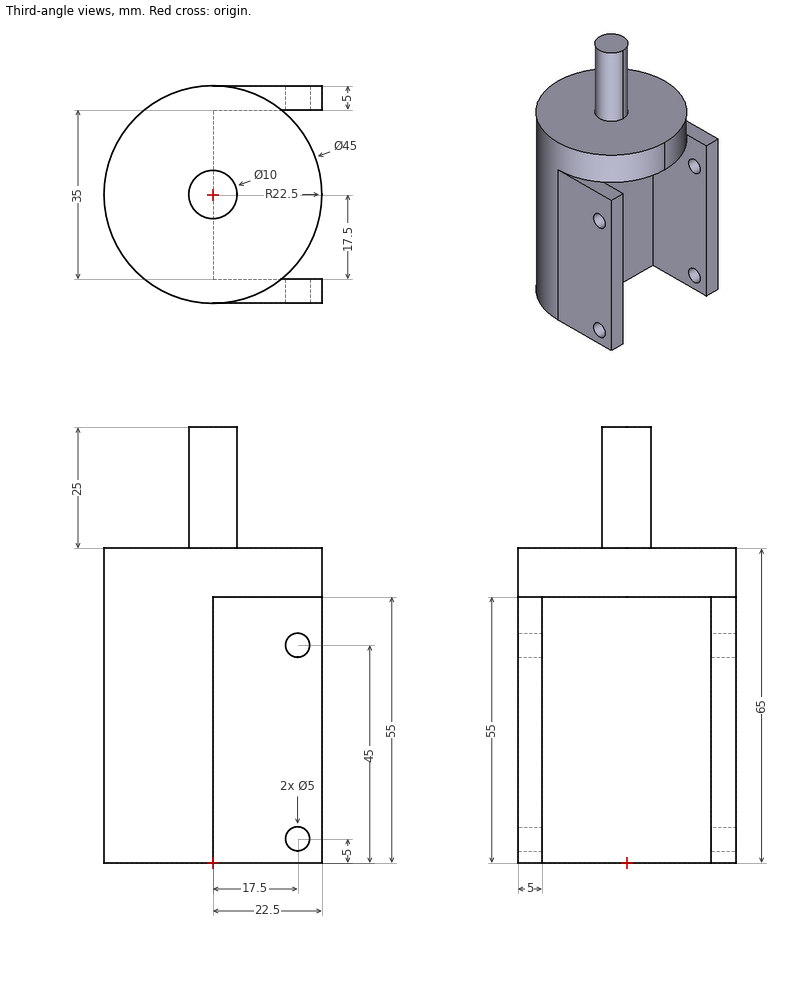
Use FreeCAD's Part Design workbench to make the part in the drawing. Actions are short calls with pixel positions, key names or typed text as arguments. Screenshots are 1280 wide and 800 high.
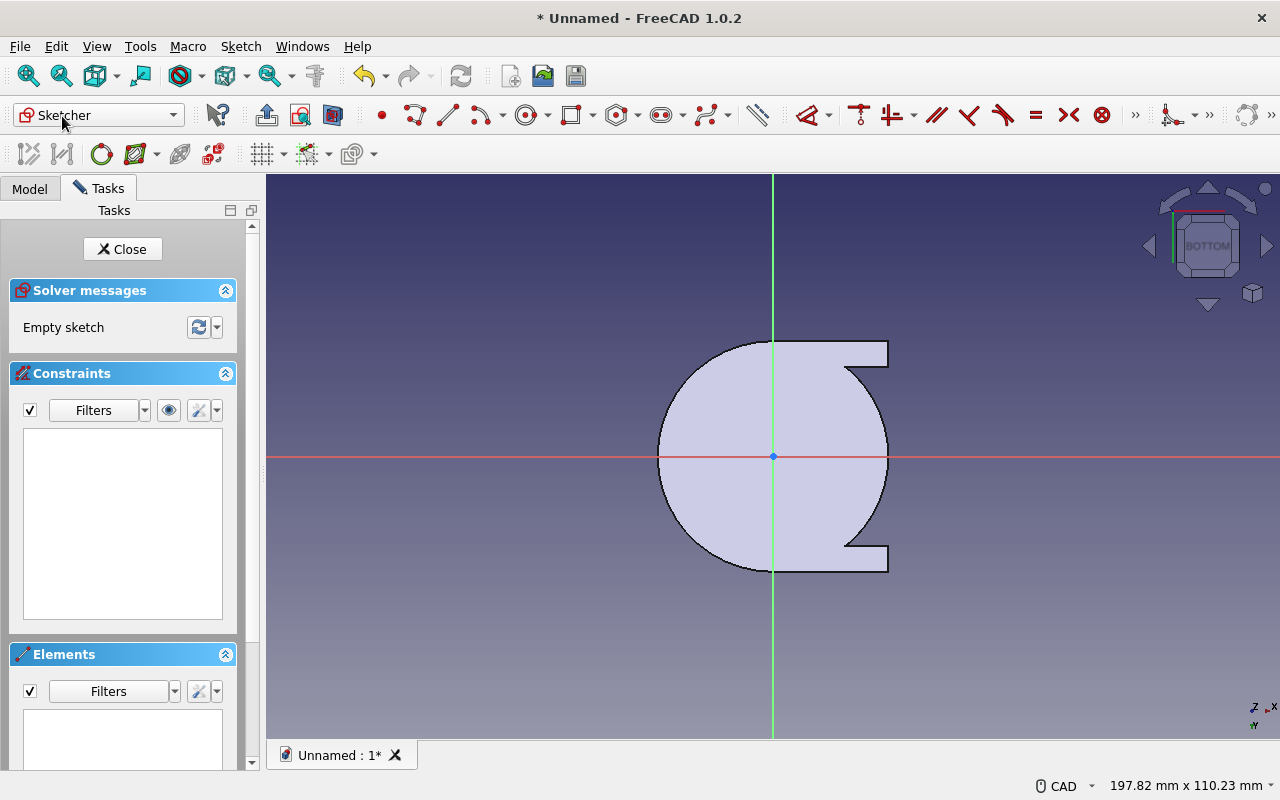
scroll(984, 456, up, 3)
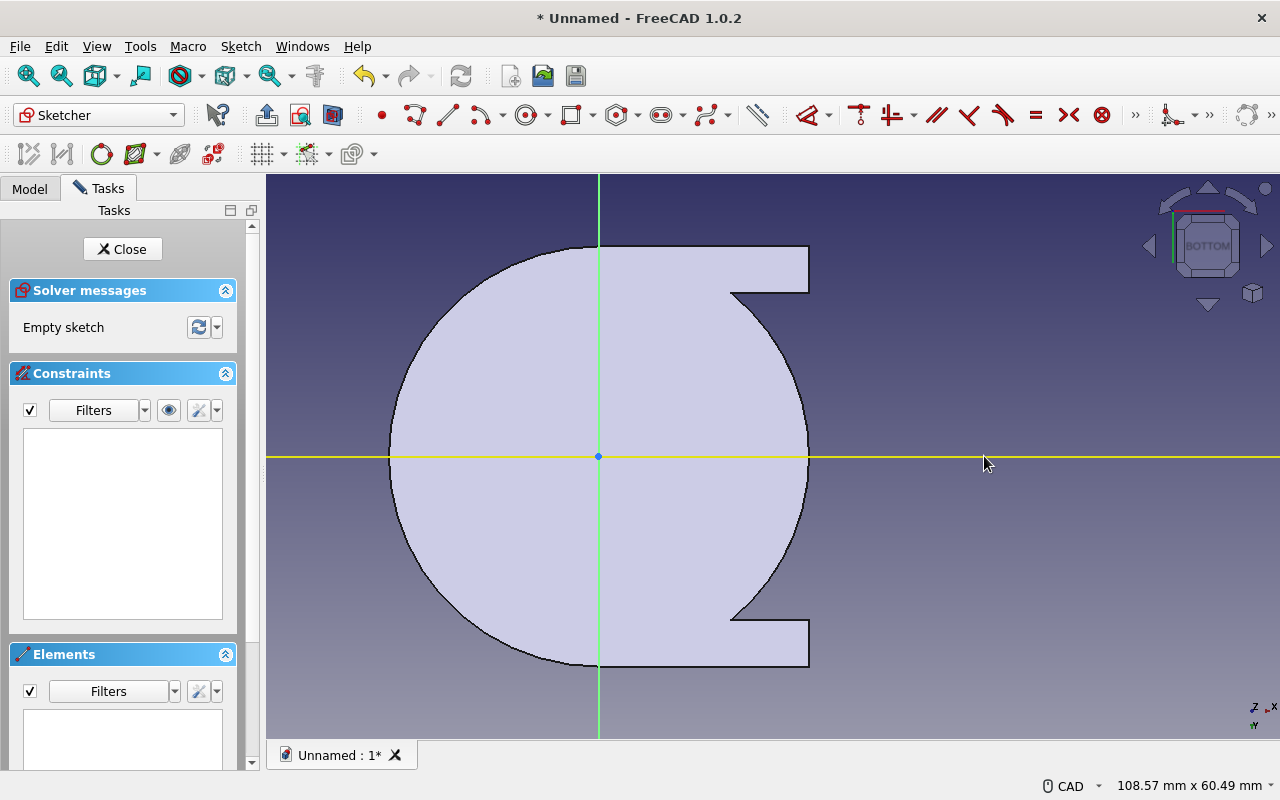
click(415, 116)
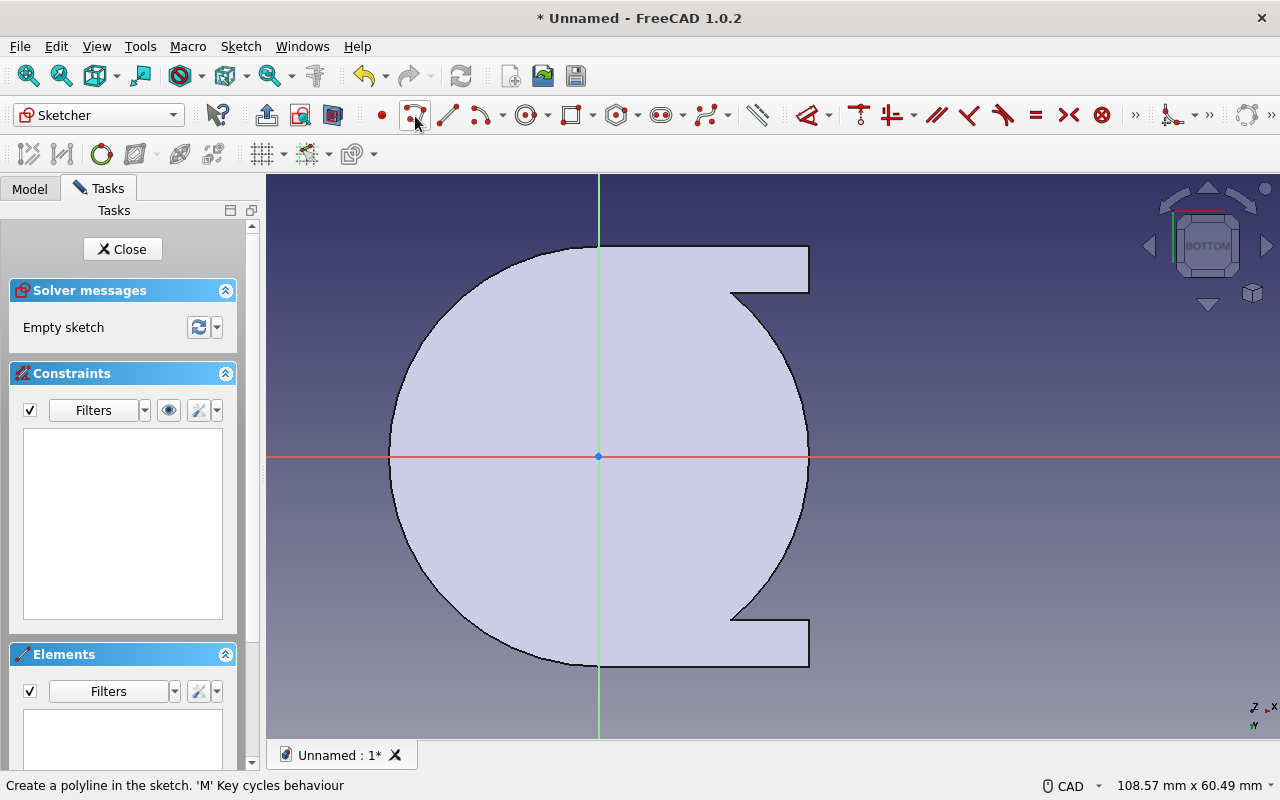
click(731, 293)
click(599, 293)
click(608, 620)
click(731, 620)
right_click(731, 620)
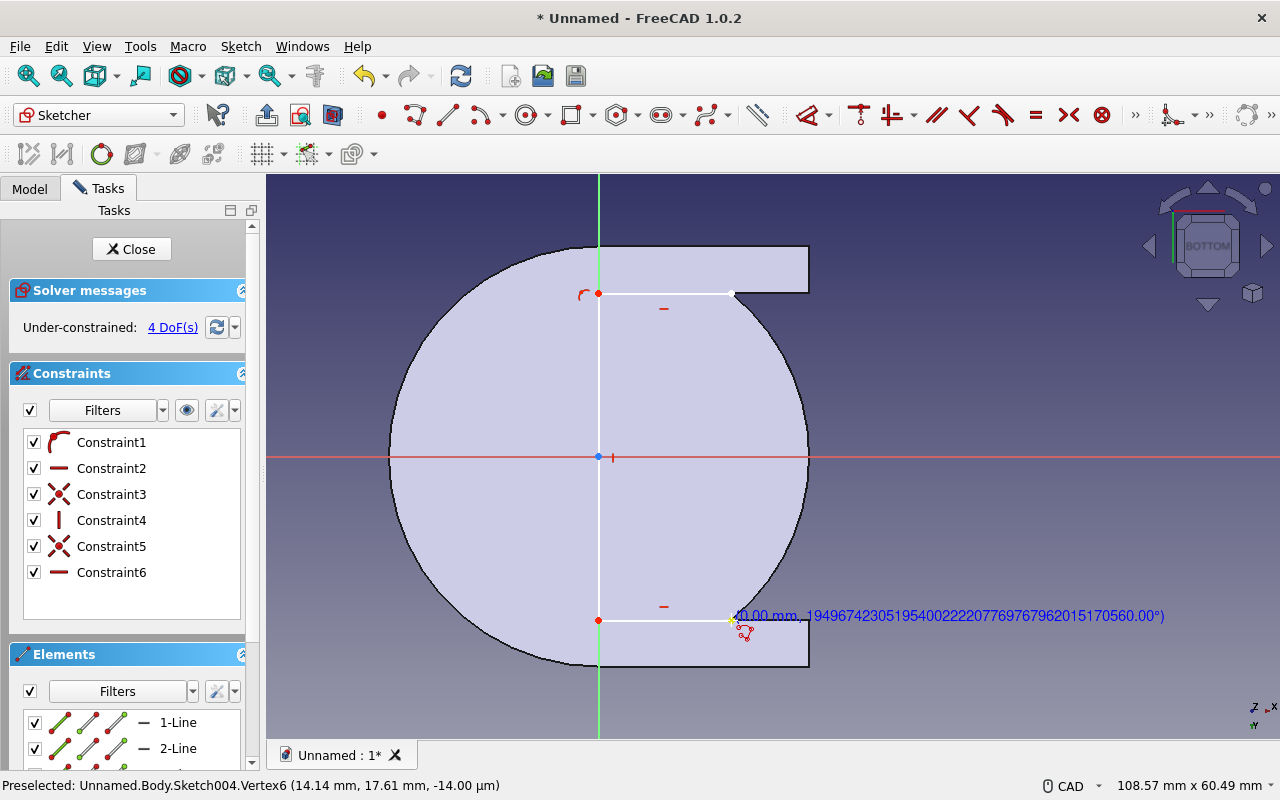
key(g)
key(3)
key(a)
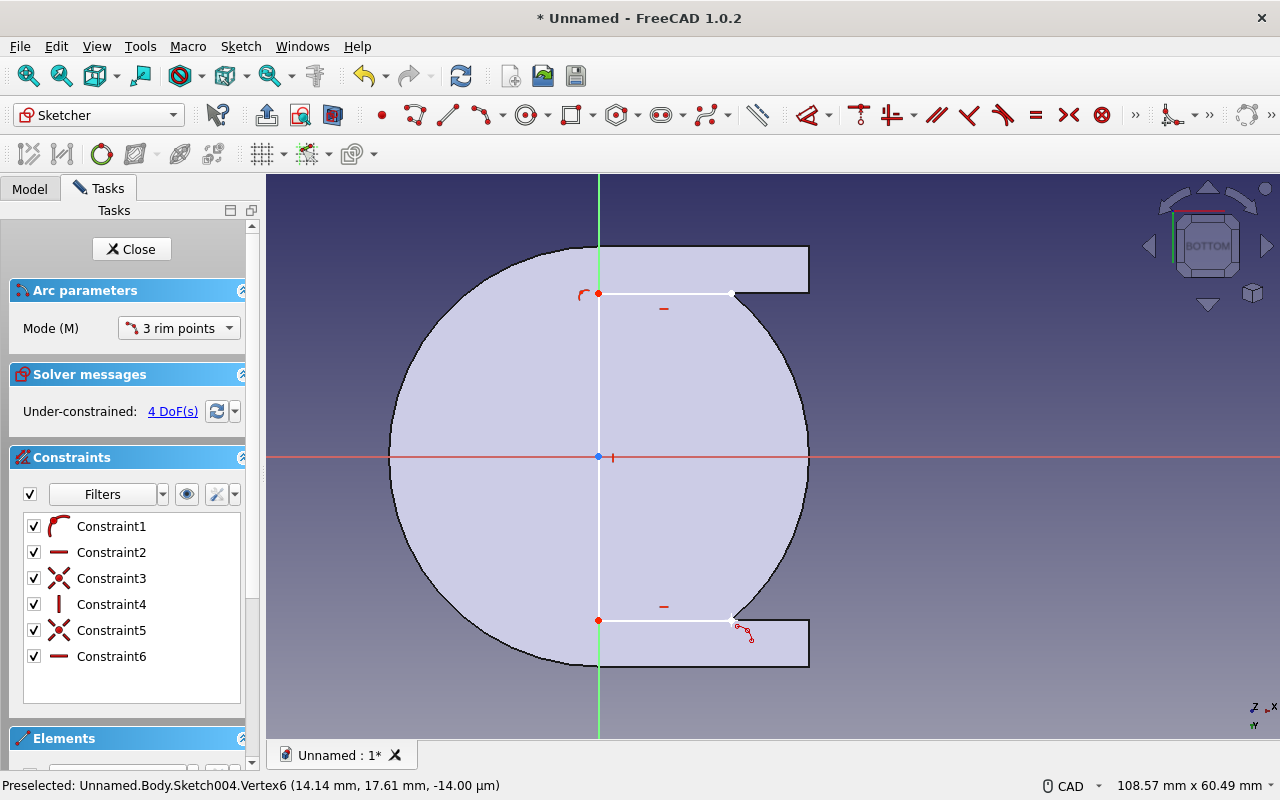
click(731, 621)
click(731, 294)
click(806, 494)
key(Escape)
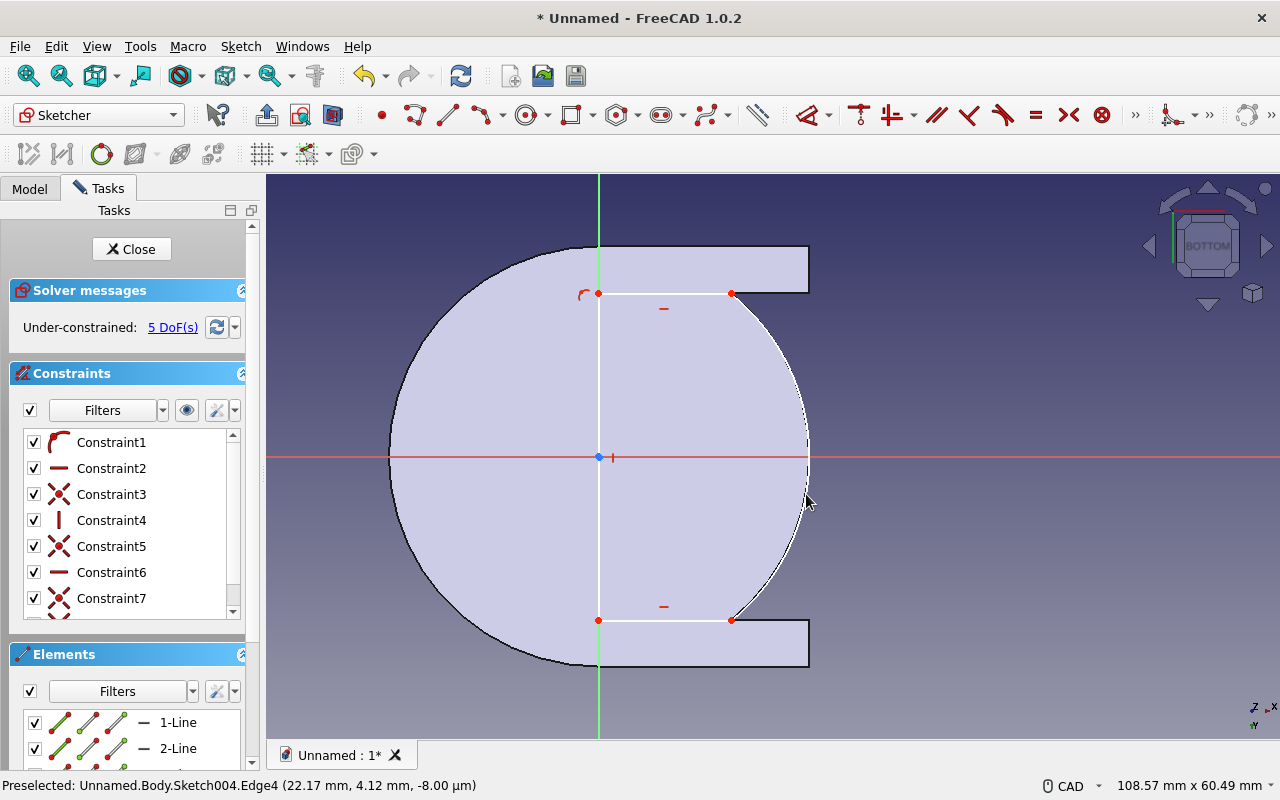
drag(589, 446, 610, 468)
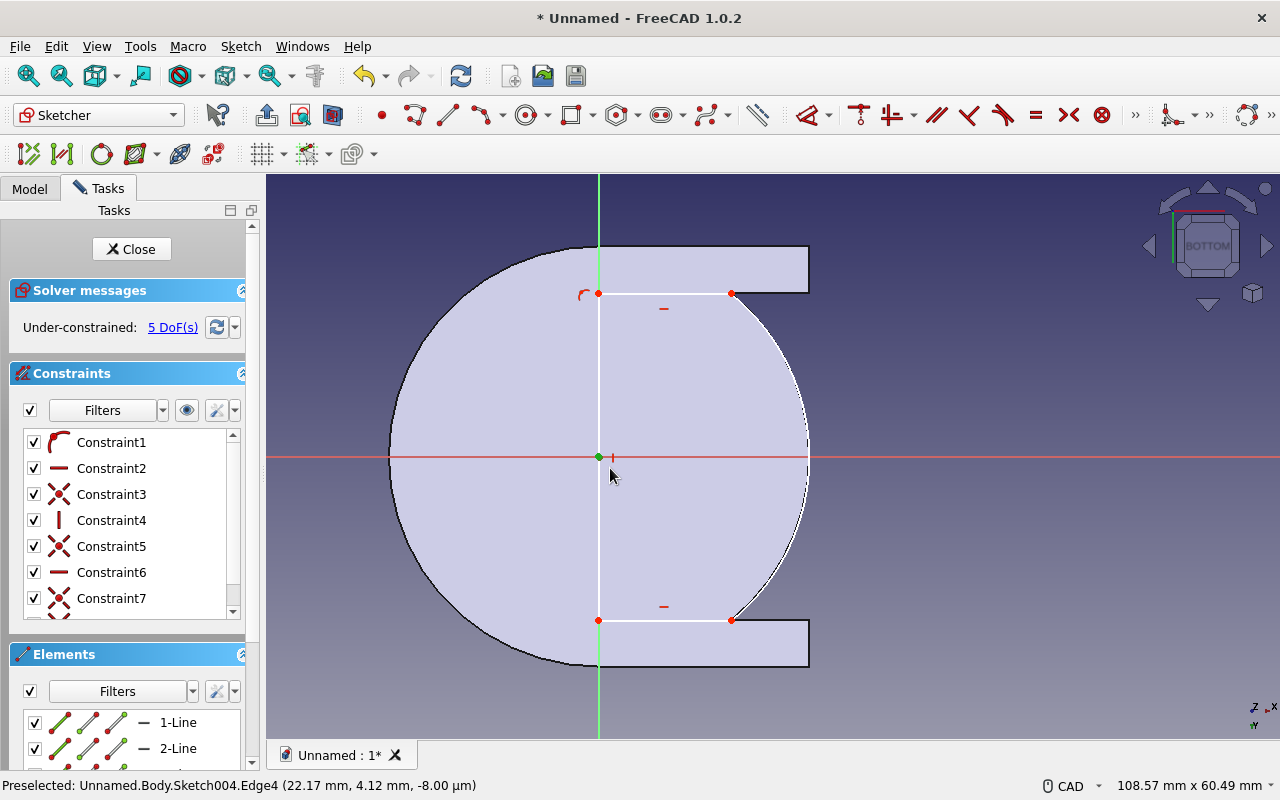
click(859, 116)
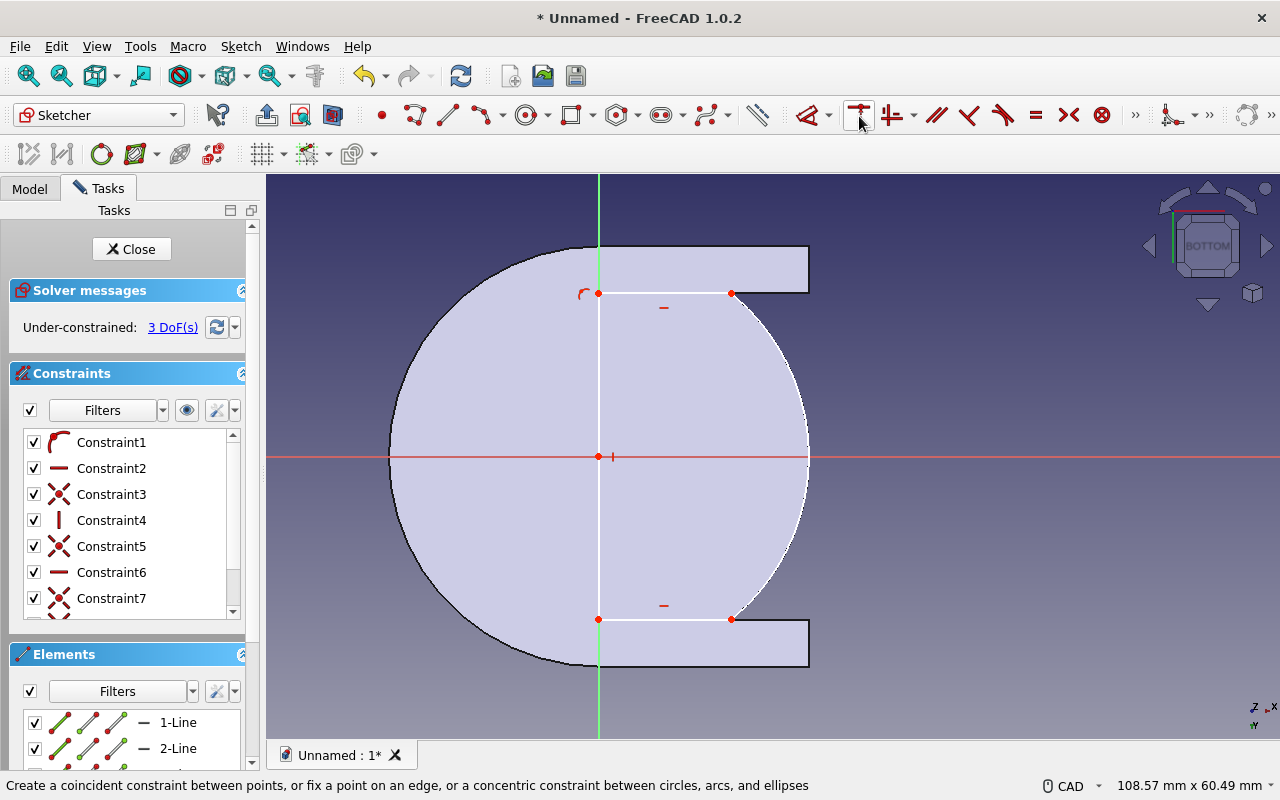
click(806, 116)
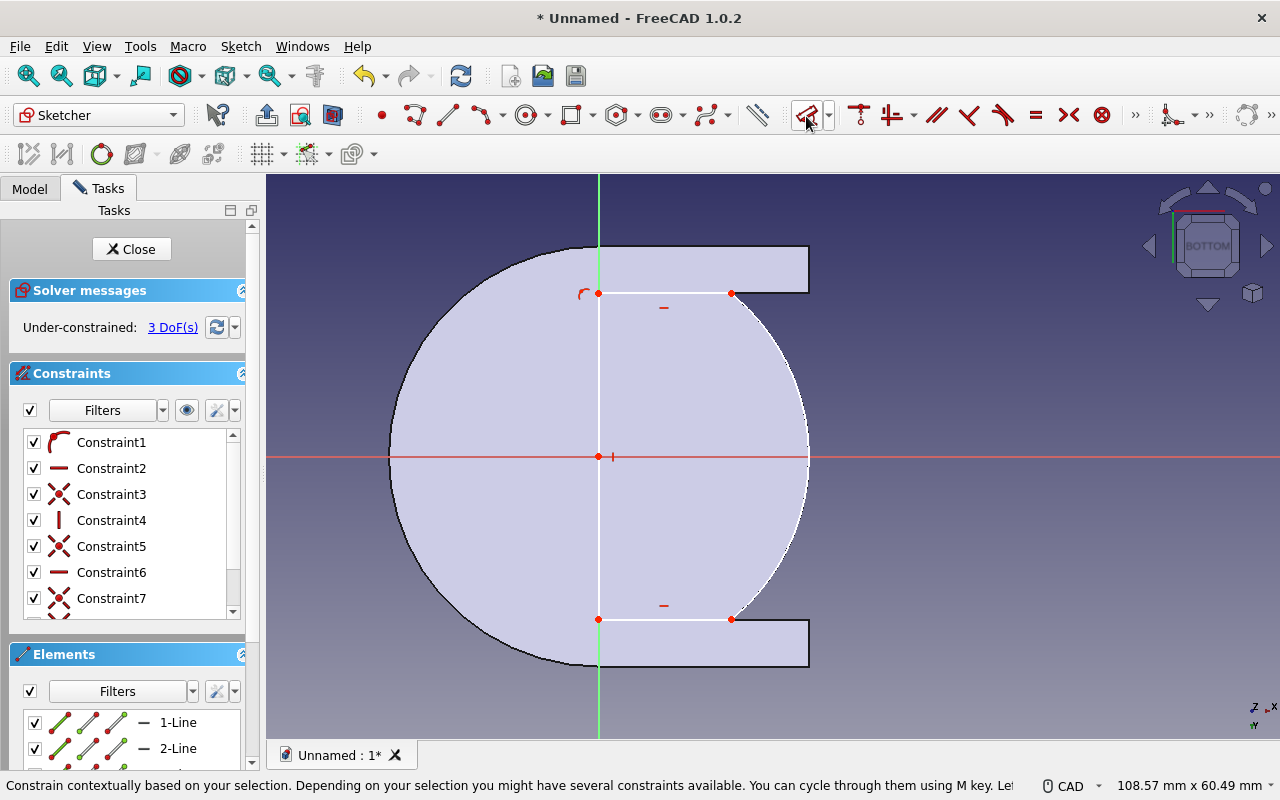
click(796, 530)
click(826, 541)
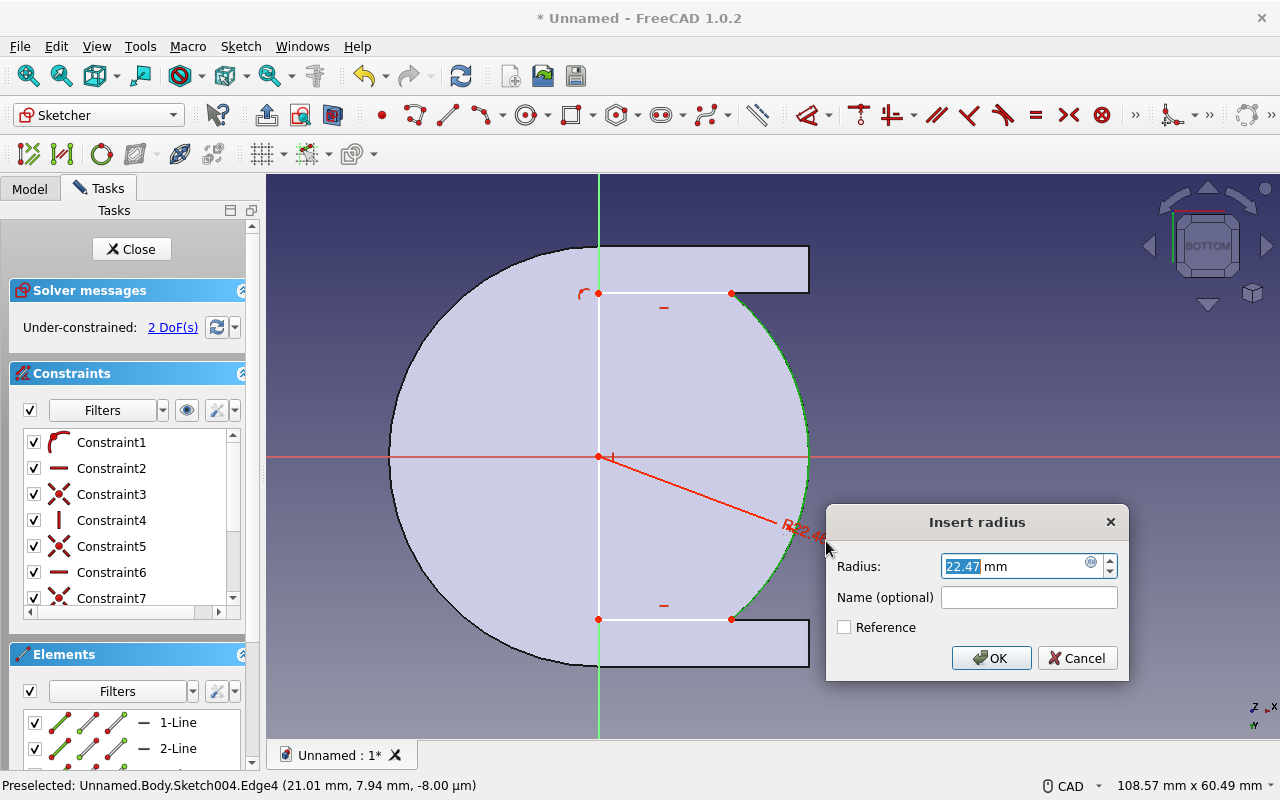
text(22.5)
key(Return)